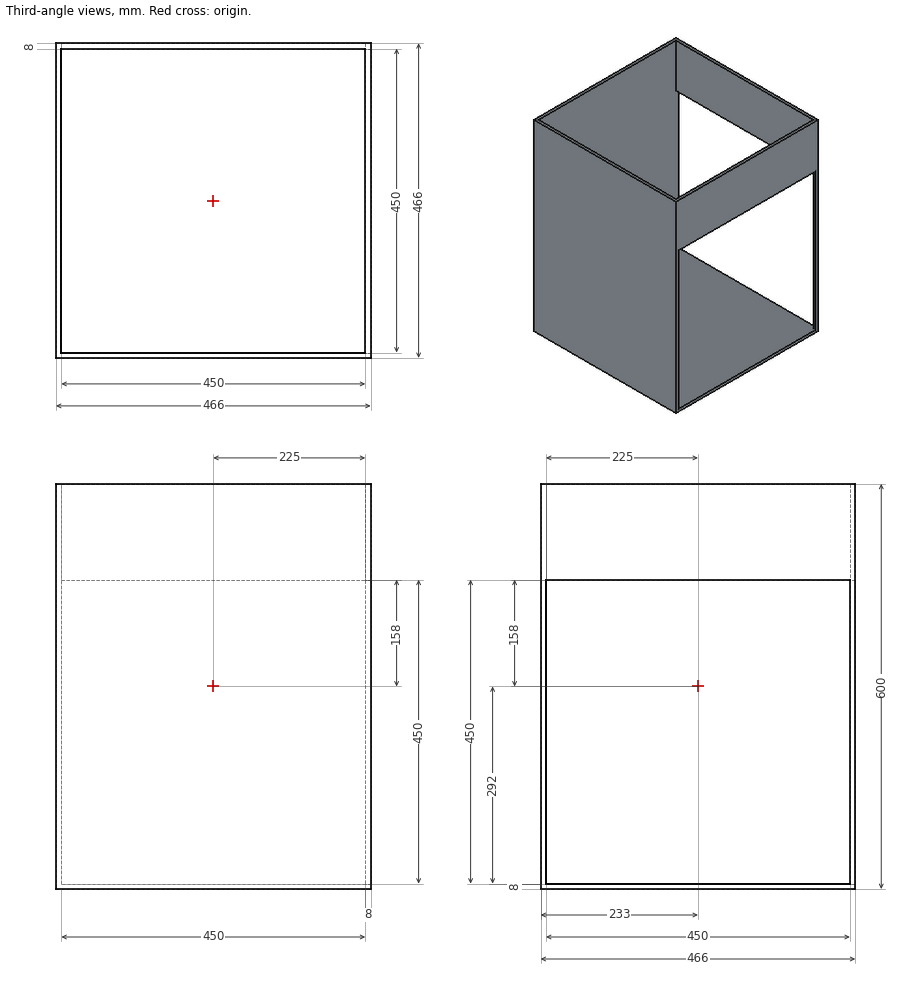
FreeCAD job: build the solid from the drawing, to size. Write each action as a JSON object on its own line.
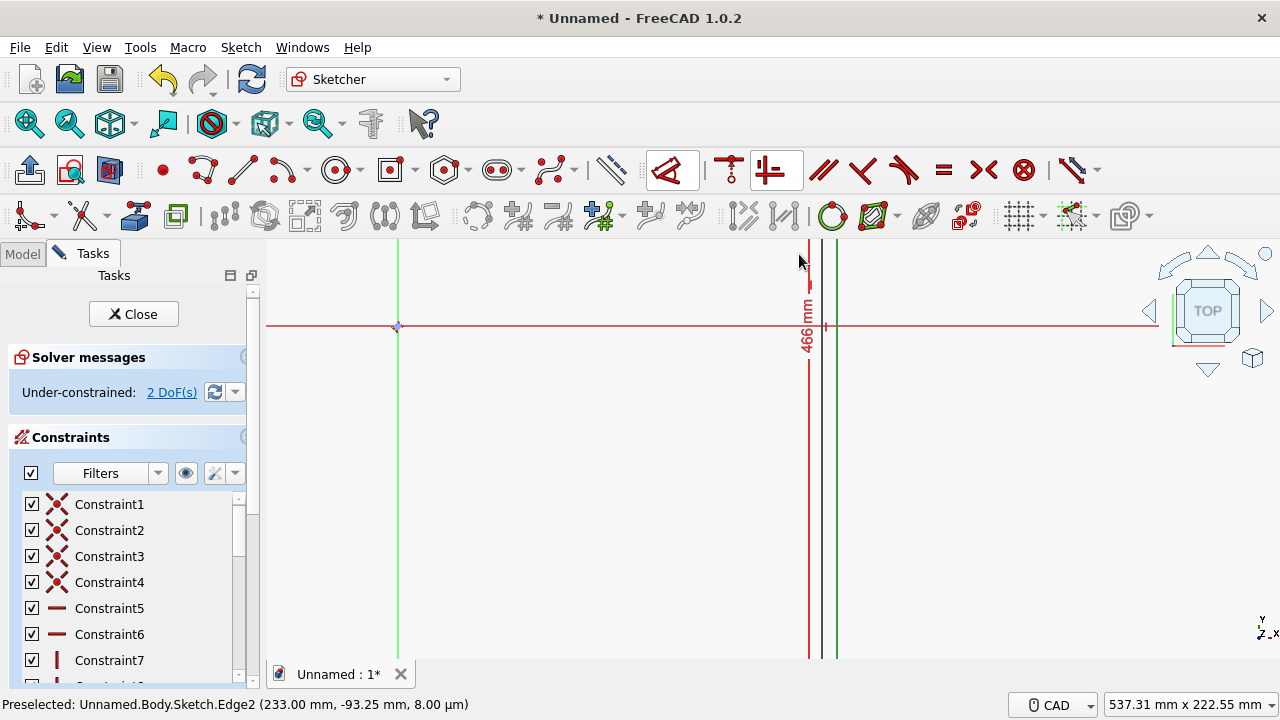
{"action": "scroll", "coordinate": [837, 502], "scroll_direction": "down", "scroll_amount": 6}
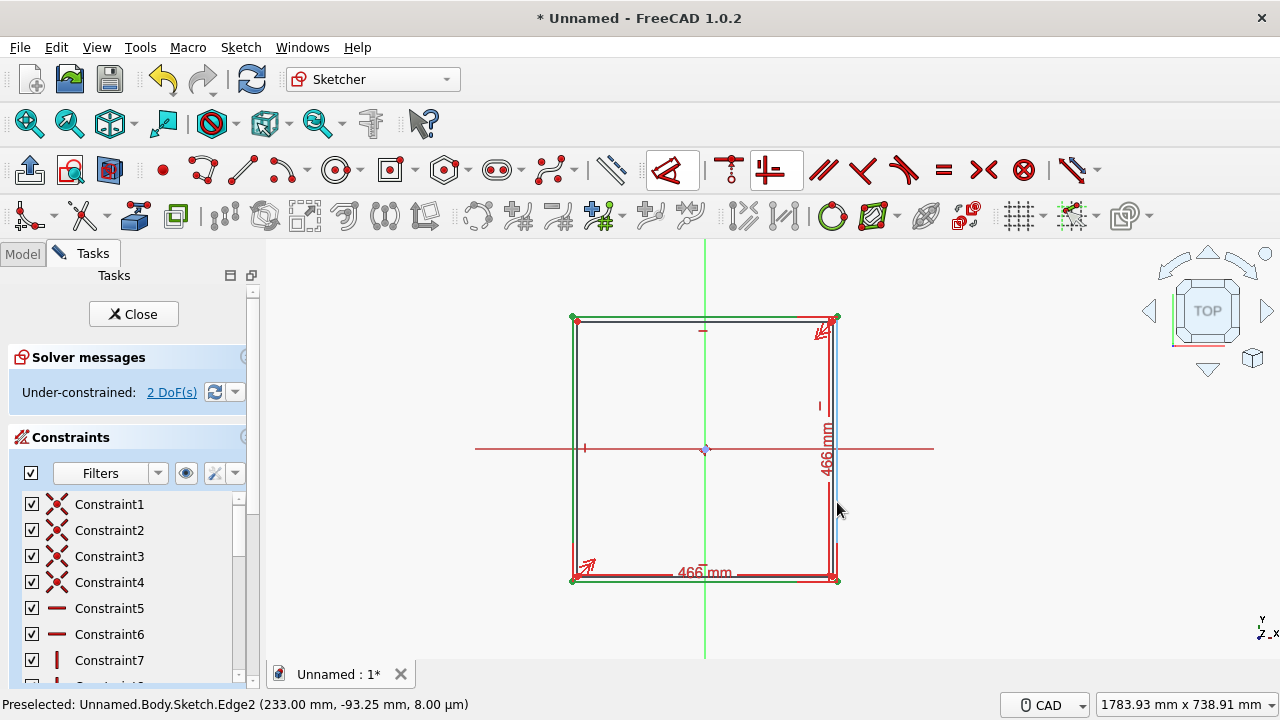
{"action": "scroll", "coordinate": [654, 577], "scroll_direction": "up", "scroll_amount": 6}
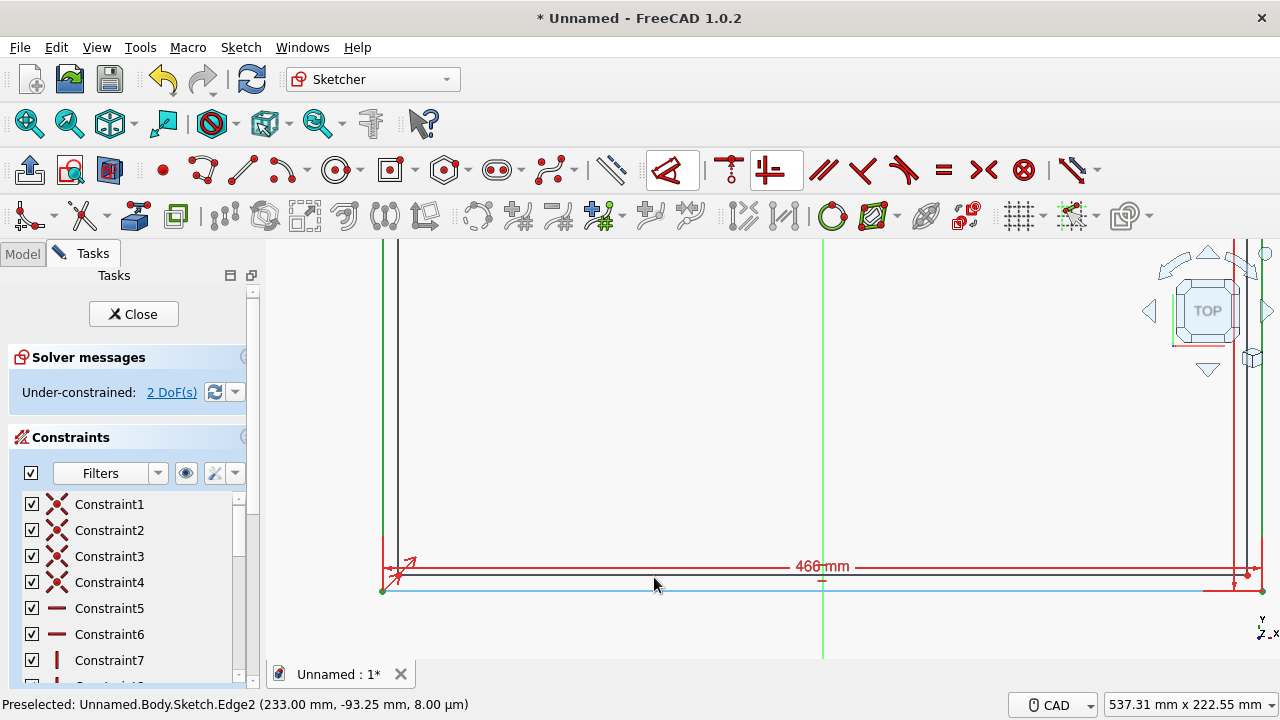
{"action": "left_click", "coordinate": [653, 575]}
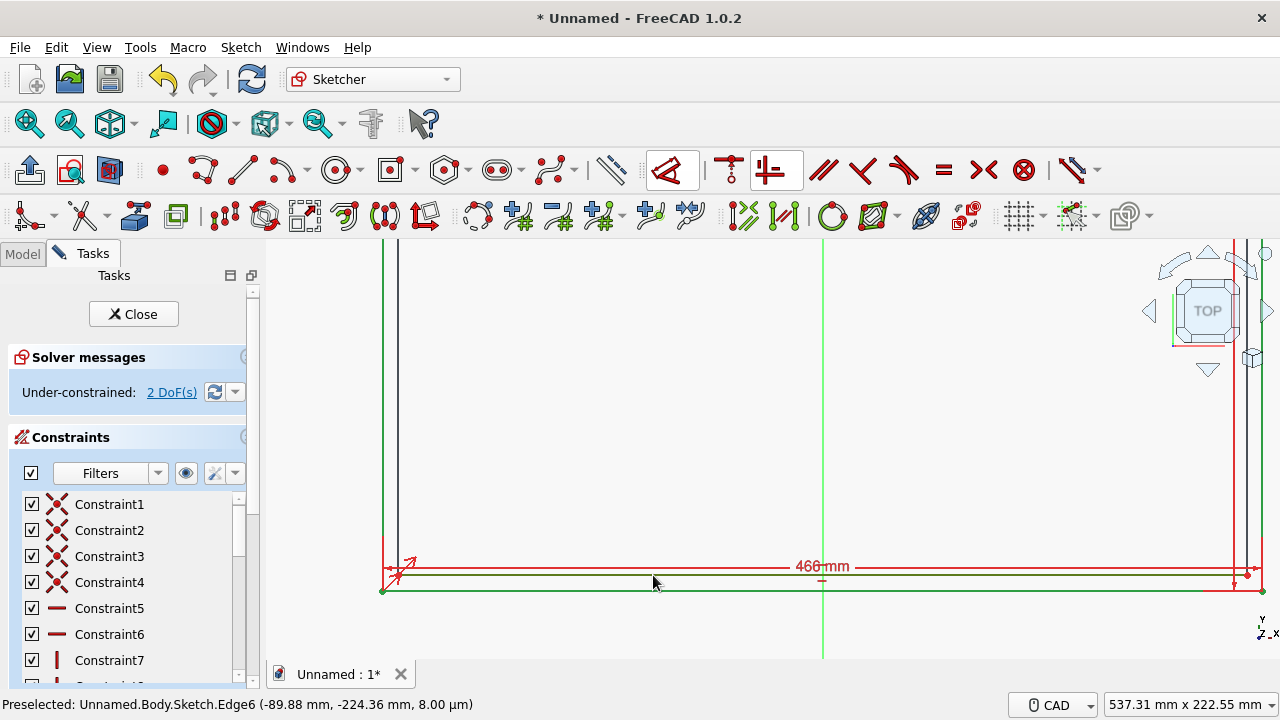
{"action": "key", "text": "l"}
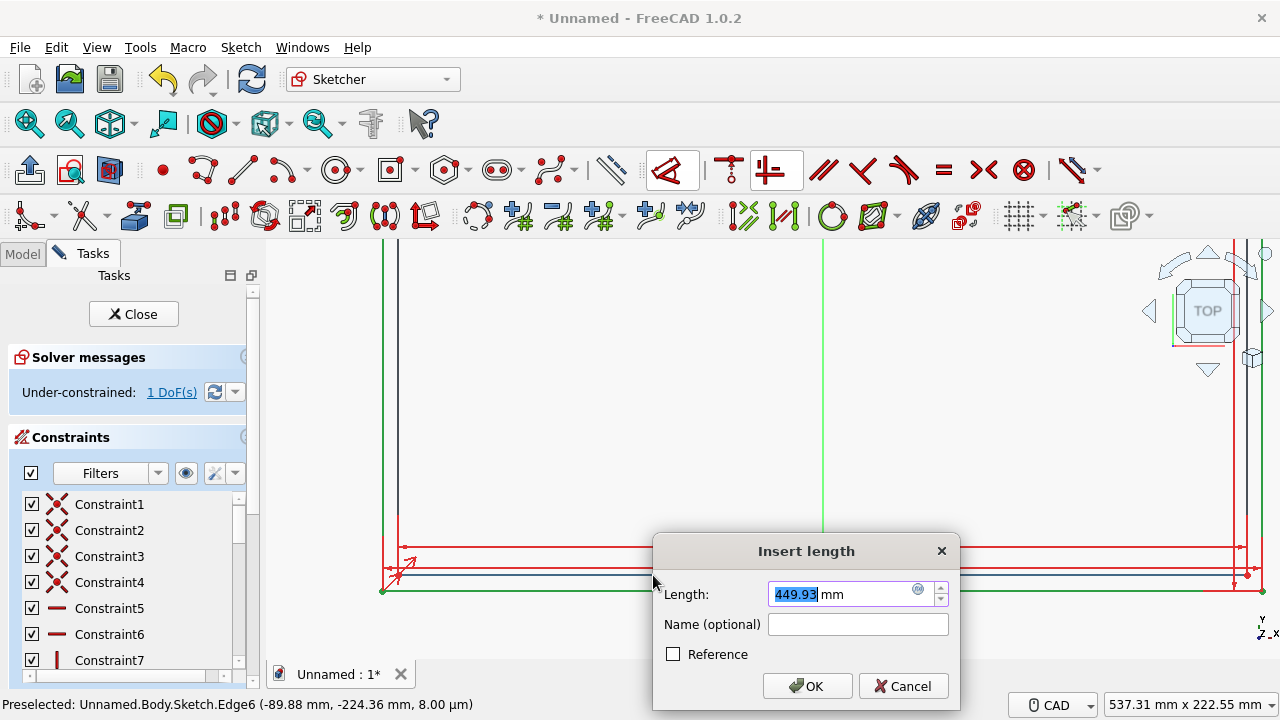
{"action": "type", "text": "450"}
{"action": "key", "text": "Return"}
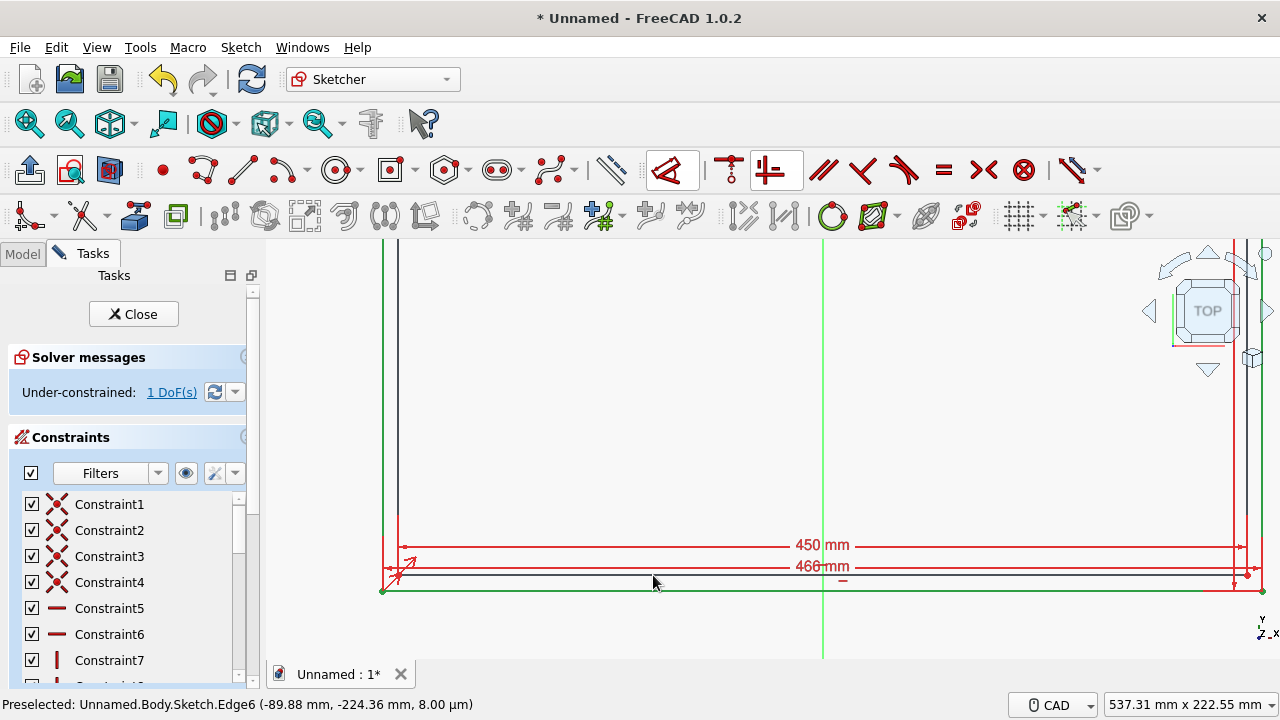
{"action": "scroll", "coordinate": [654, 577], "scroll_direction": "down", "scroll_amount": 6}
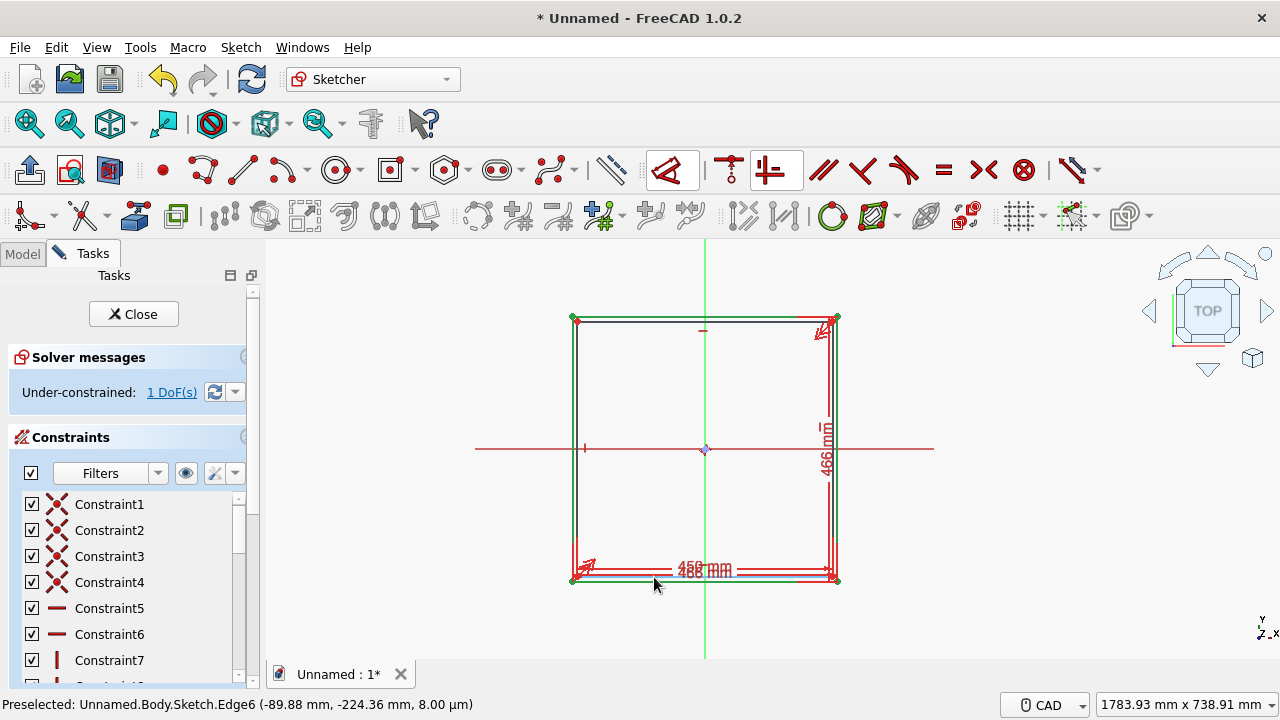
{"action": "scroll", "coordinate": [833, 500], "scroll_direction": "up", "scroll_amount": 6}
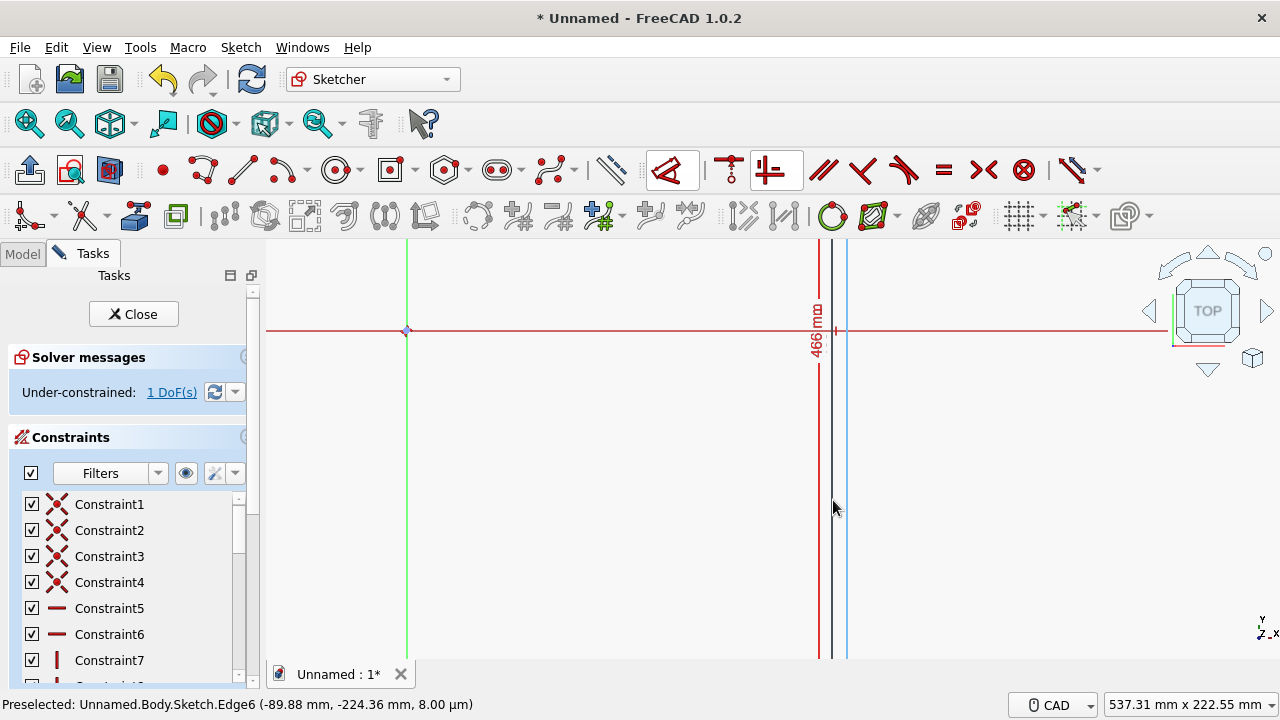
{"action": "left_click", "coordinate": [832, 500]}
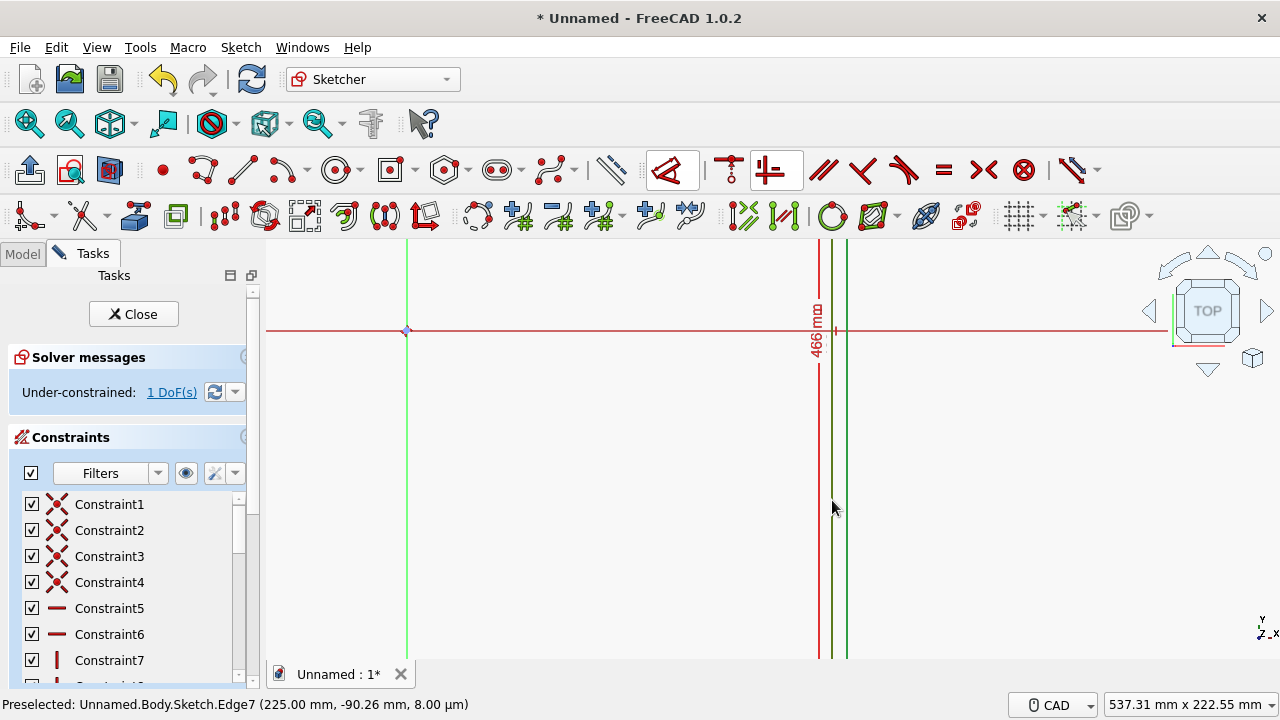
{"action": "left_click", "coordinate": [694, 170]}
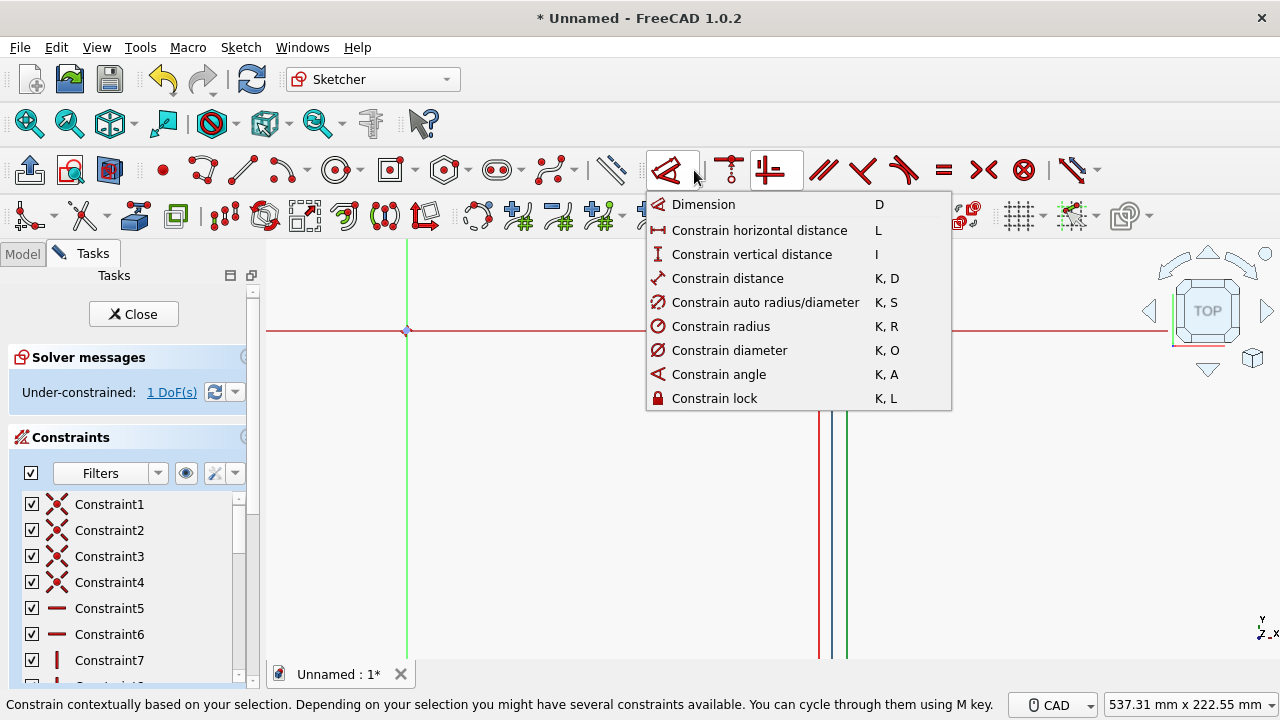
{"action": "left_click", "coordinate": [799, 254]}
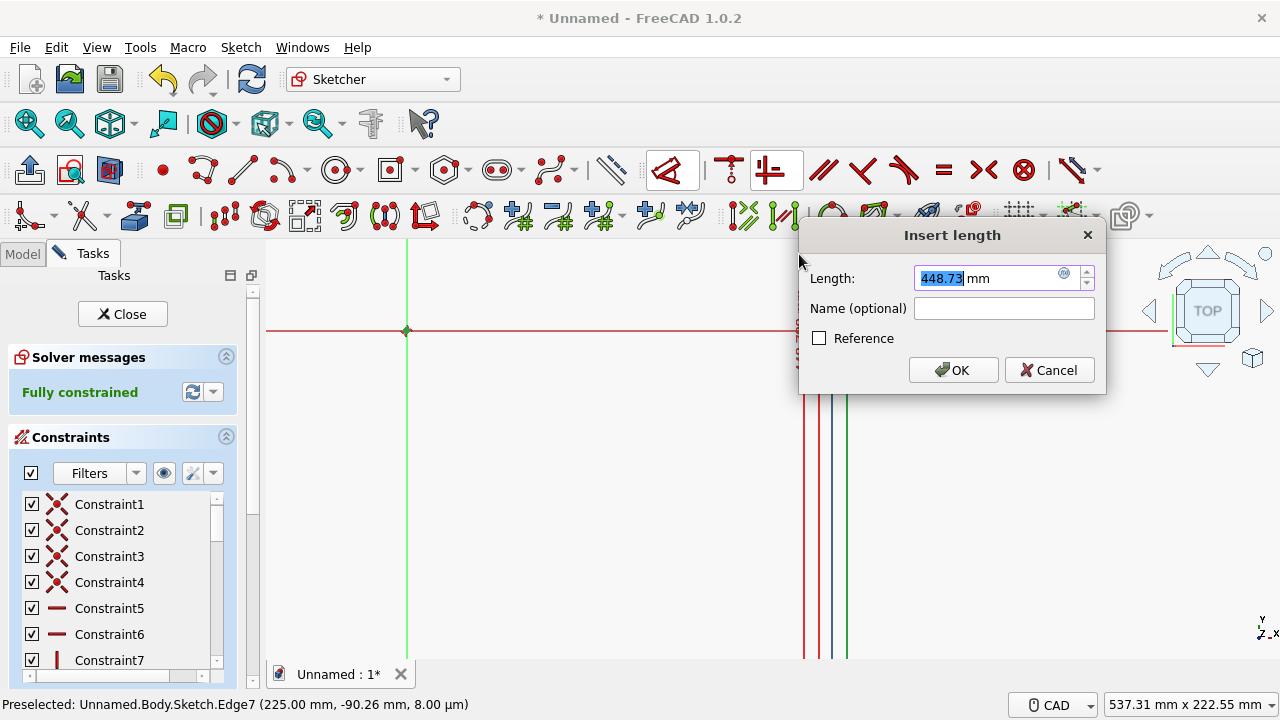
{"action": "type", "text": "450"}
{"action": "key", "text": "Return"}